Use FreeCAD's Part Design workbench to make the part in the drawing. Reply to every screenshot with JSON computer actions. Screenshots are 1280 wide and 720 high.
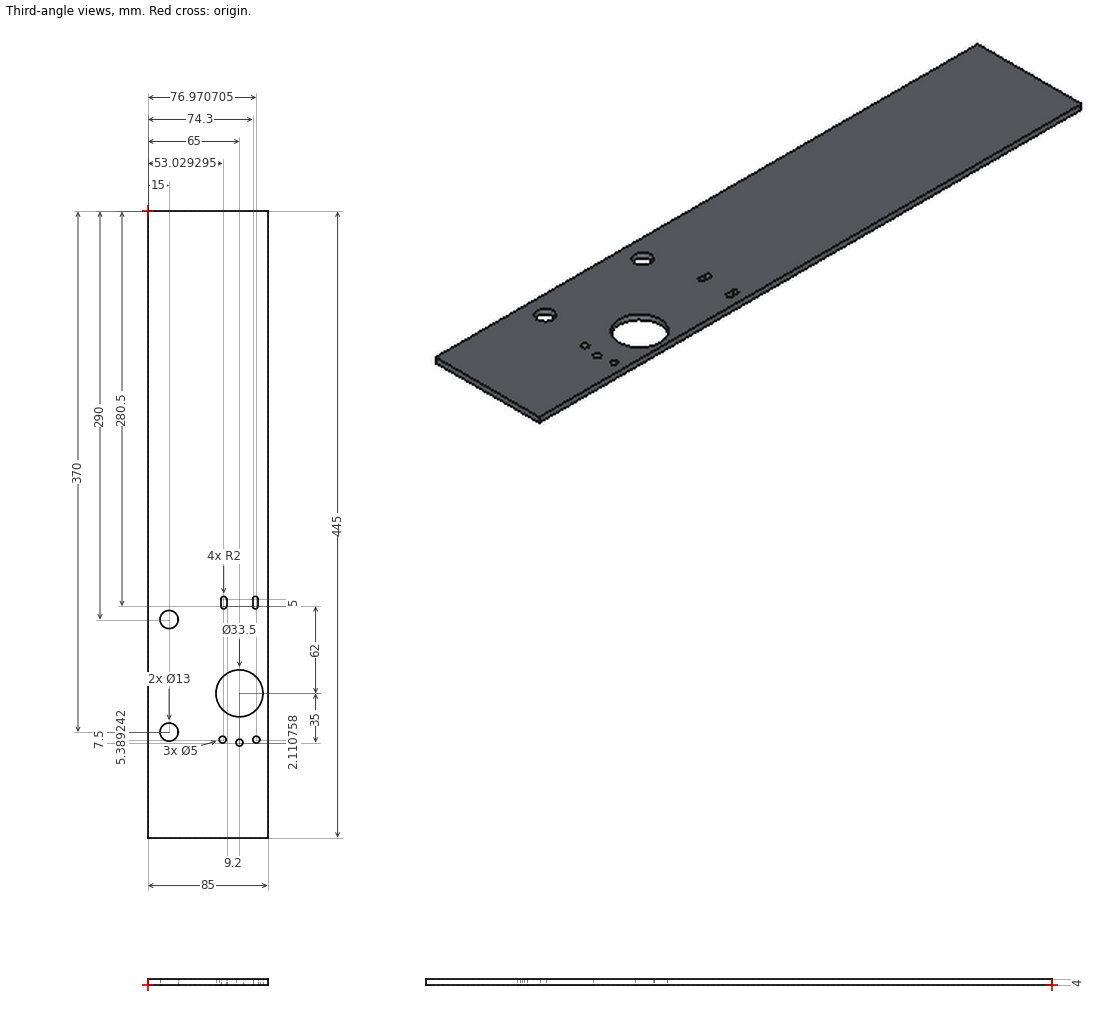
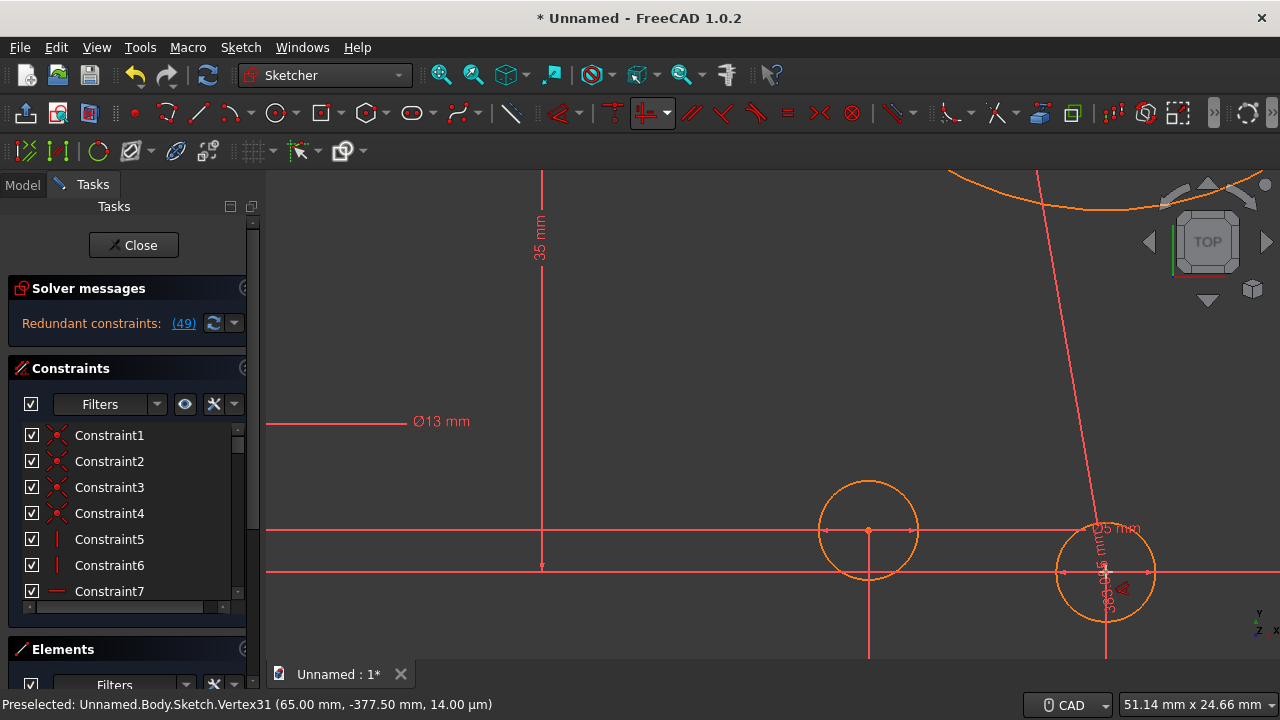
{"action": "scroll", "coordinate": [706, 538], "scroll_direction": "down", "scroll_amount": 16}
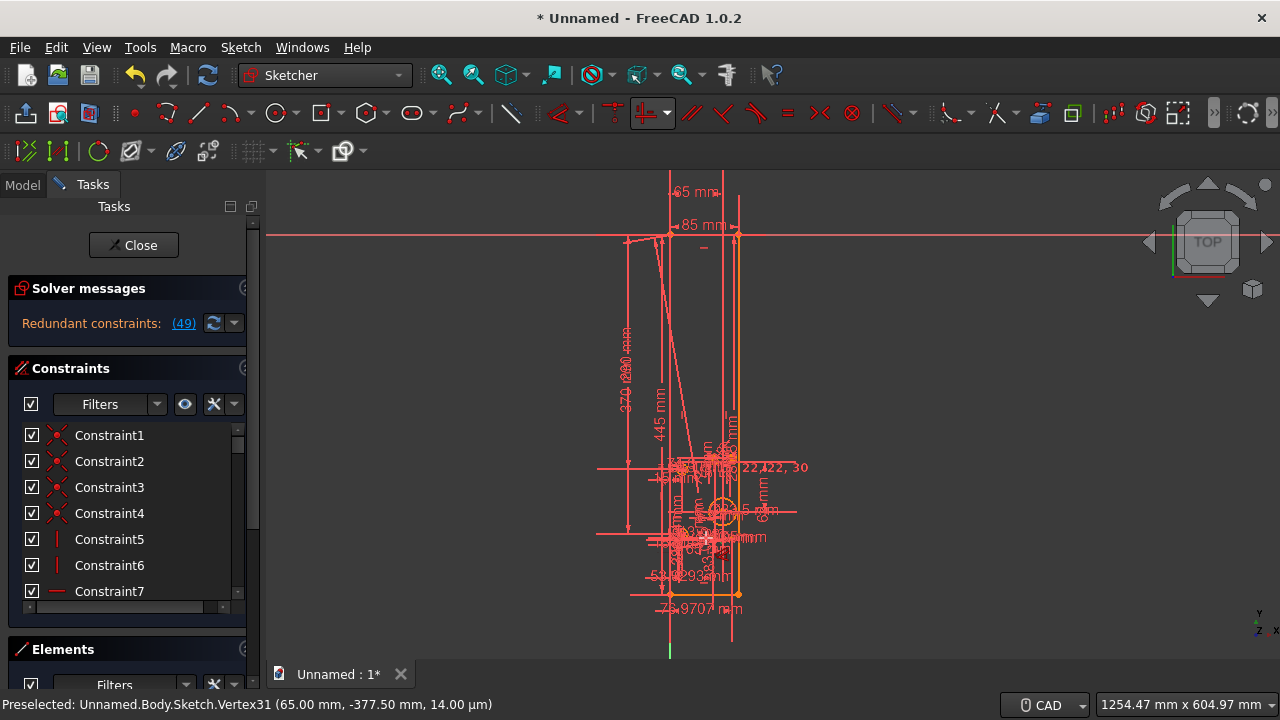
{"action": "scroll", "coordinate": [732, 539], "scroll_direction": "up", "scroll_amount": 16}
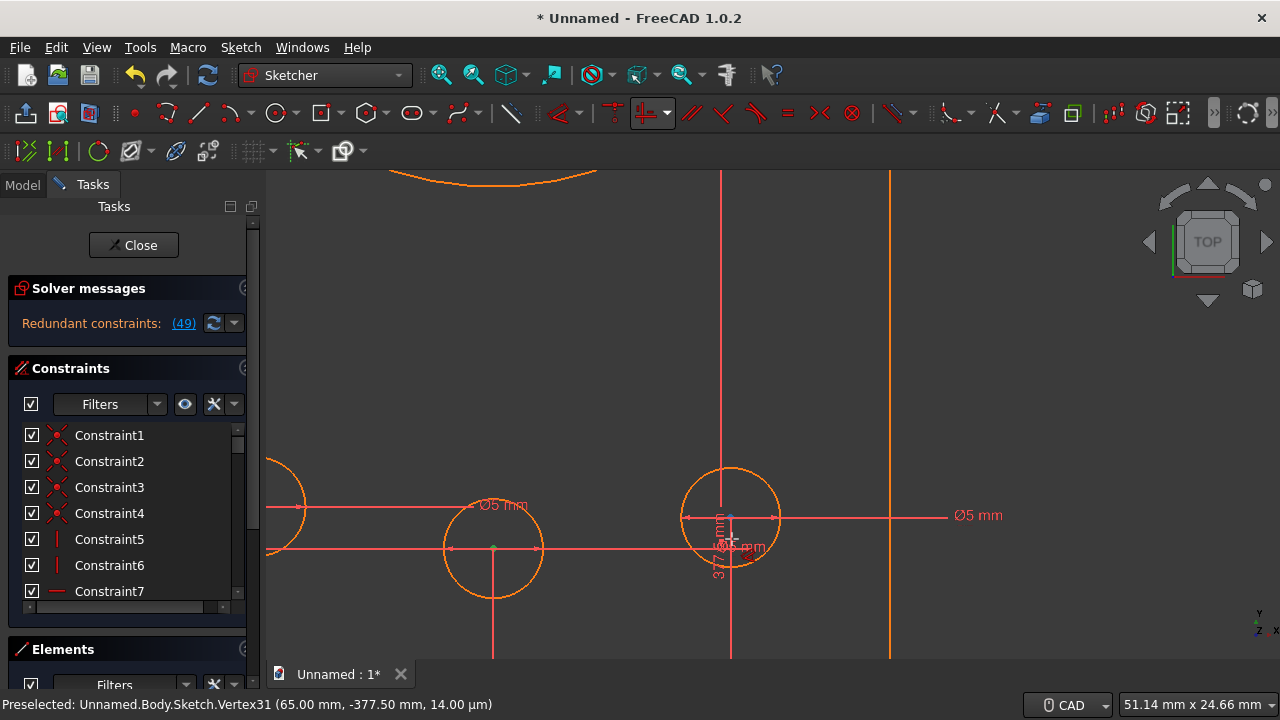
{"action": "left_click", "coordinate": [731, 518]}
{"action": "left_click", "coordinate": [765, 526]}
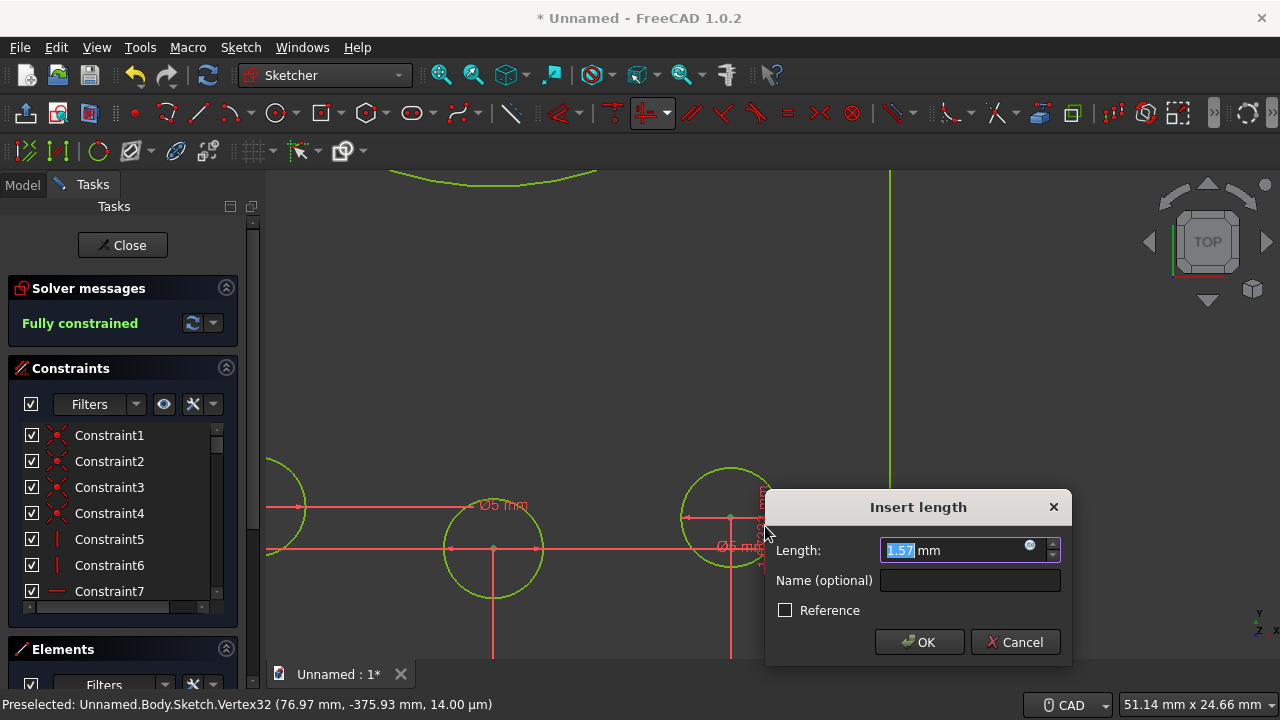
{"action": "type", "text": "2.110758"}
{"action": "key", "text": "Return"}
{"action": "key", "text": "Escape"}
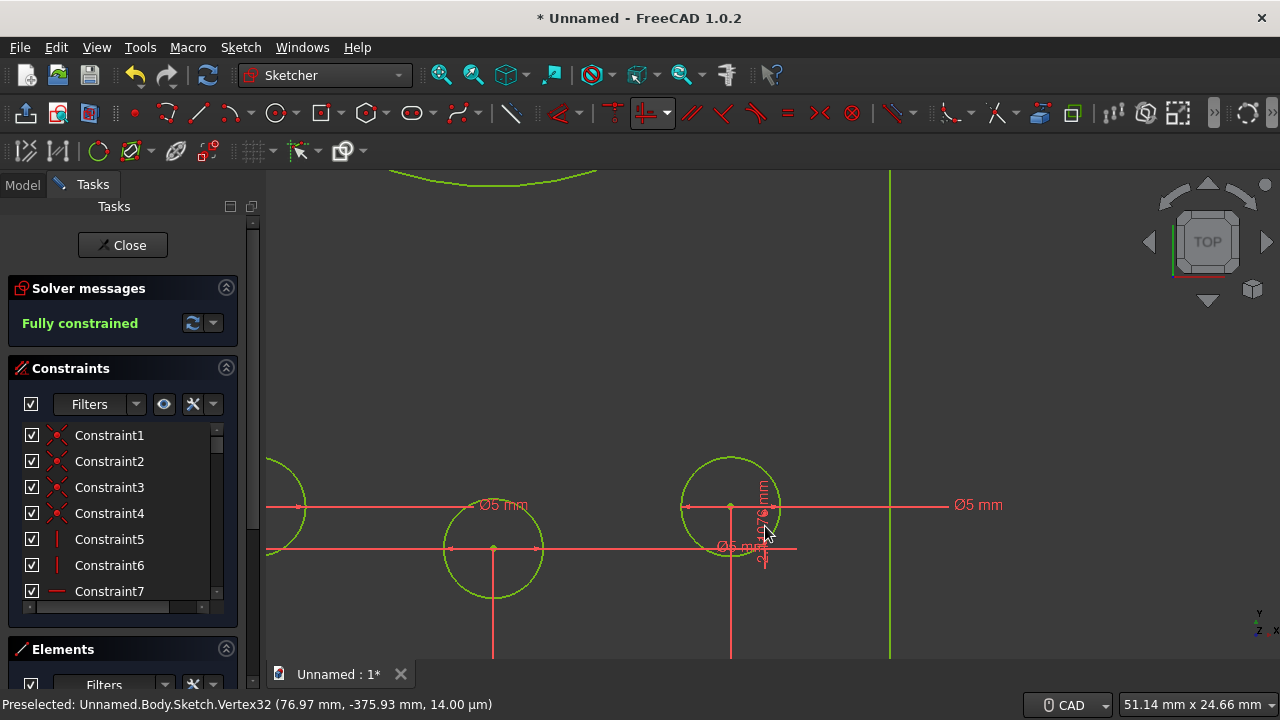
{"action": "left_click", "coordinate": [123, 245]}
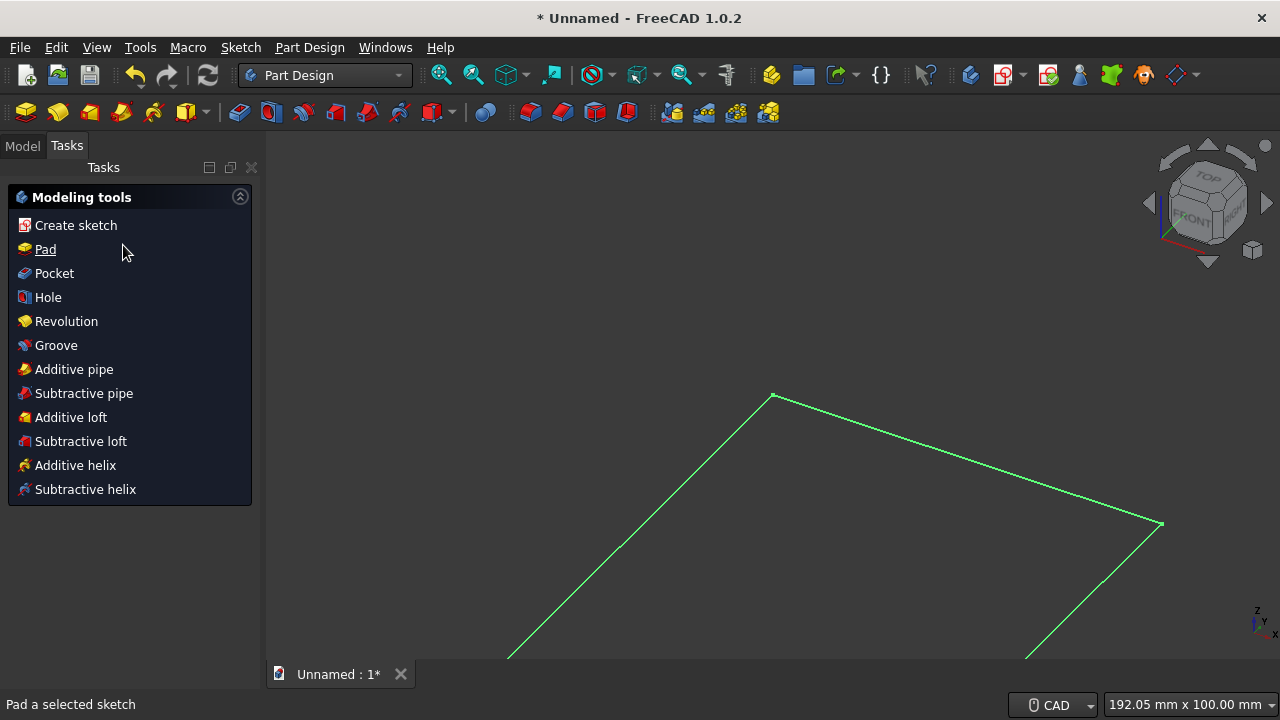
{"action": "left_click", "coordinate": [26, 112]}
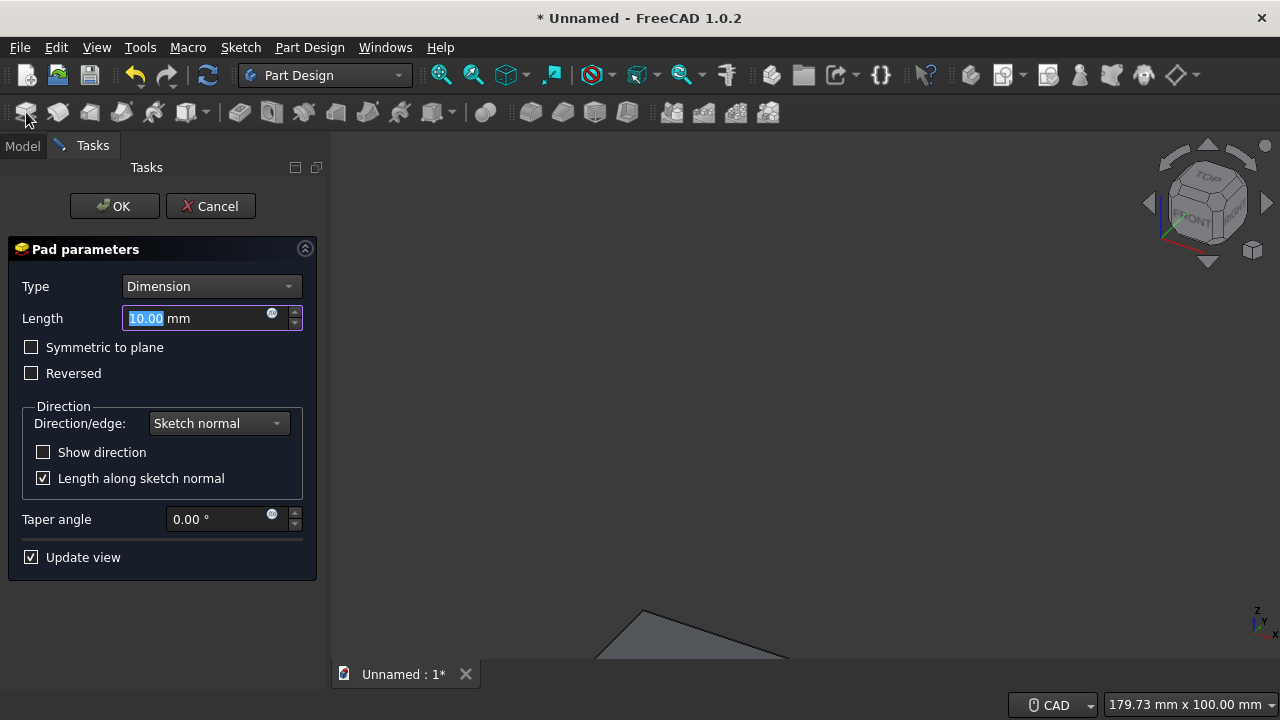
{"action": "type", "text": "4"}
{"action": "key", "text": "Tab"}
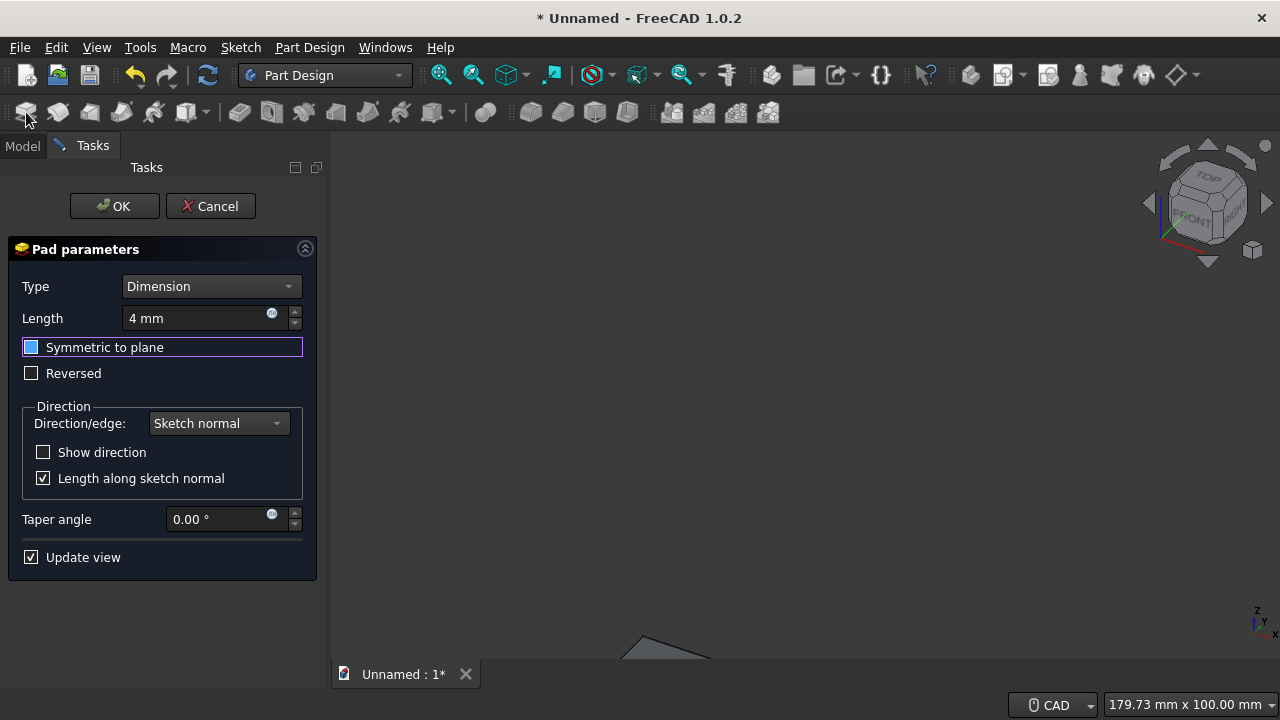
{"action": "left_click", "coordinate": [115, 206]}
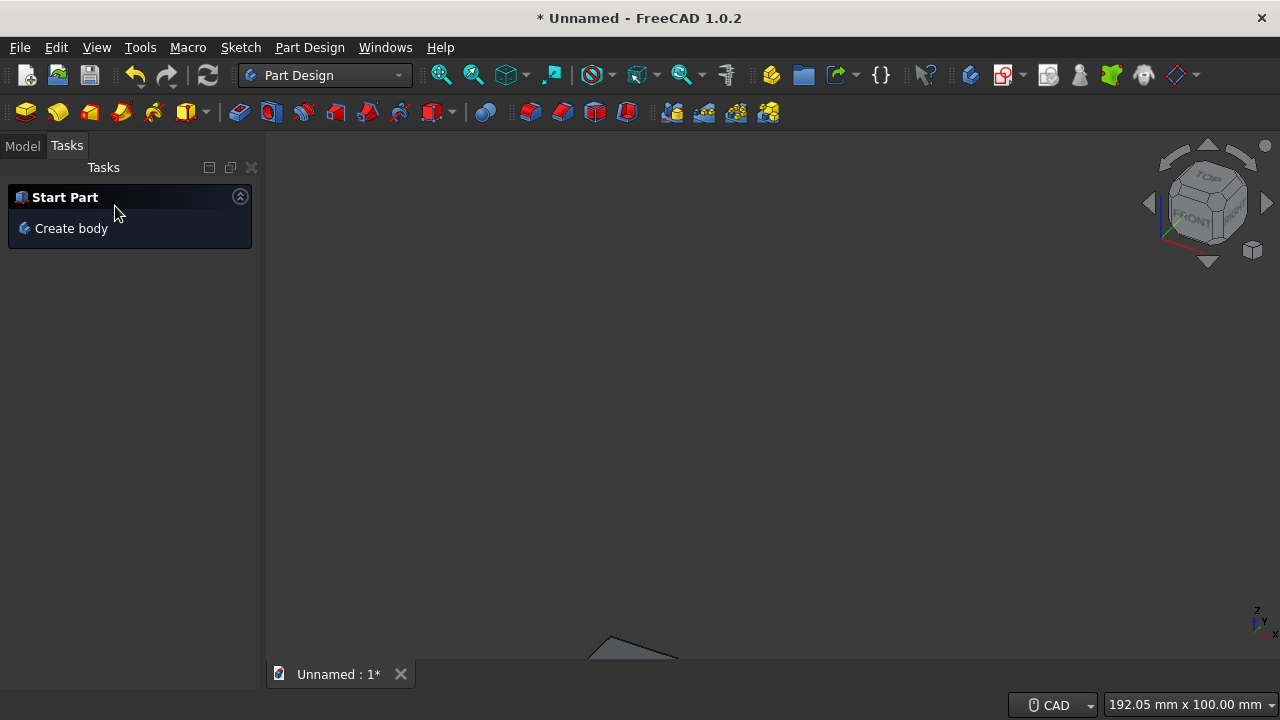
{"action": "key", "text": "0"}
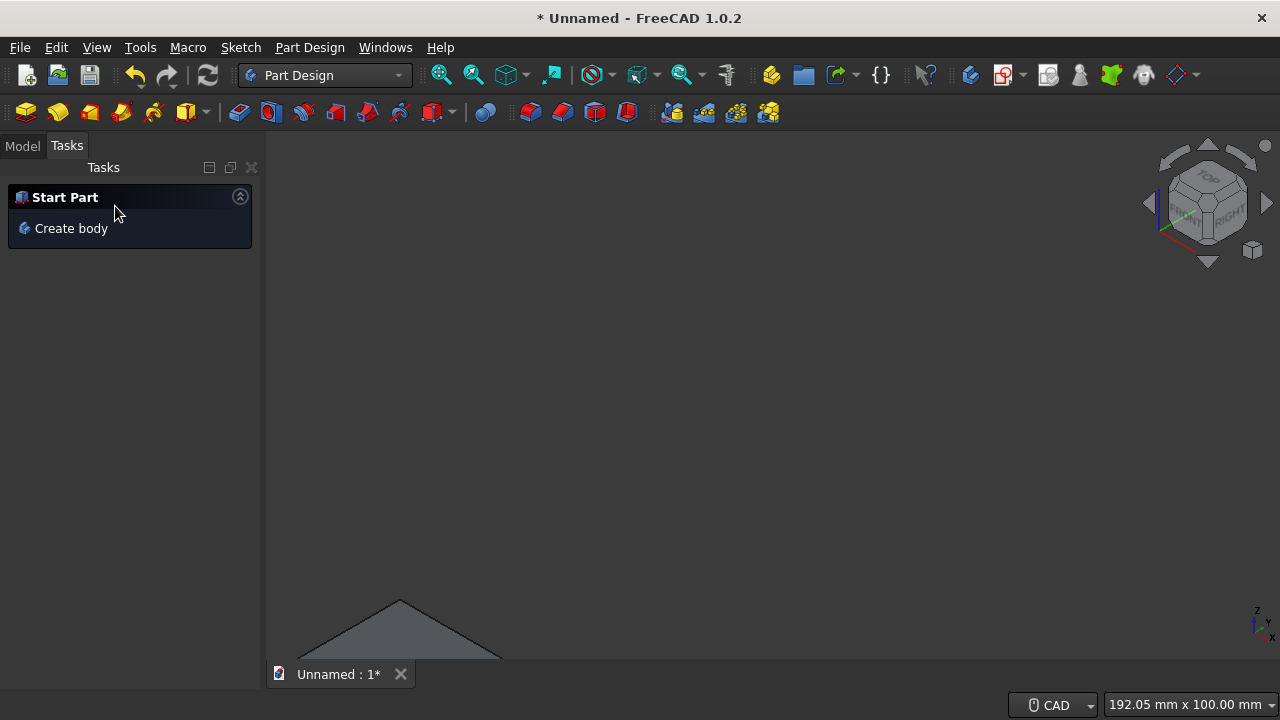
{"action": "key", "text": "v f"}